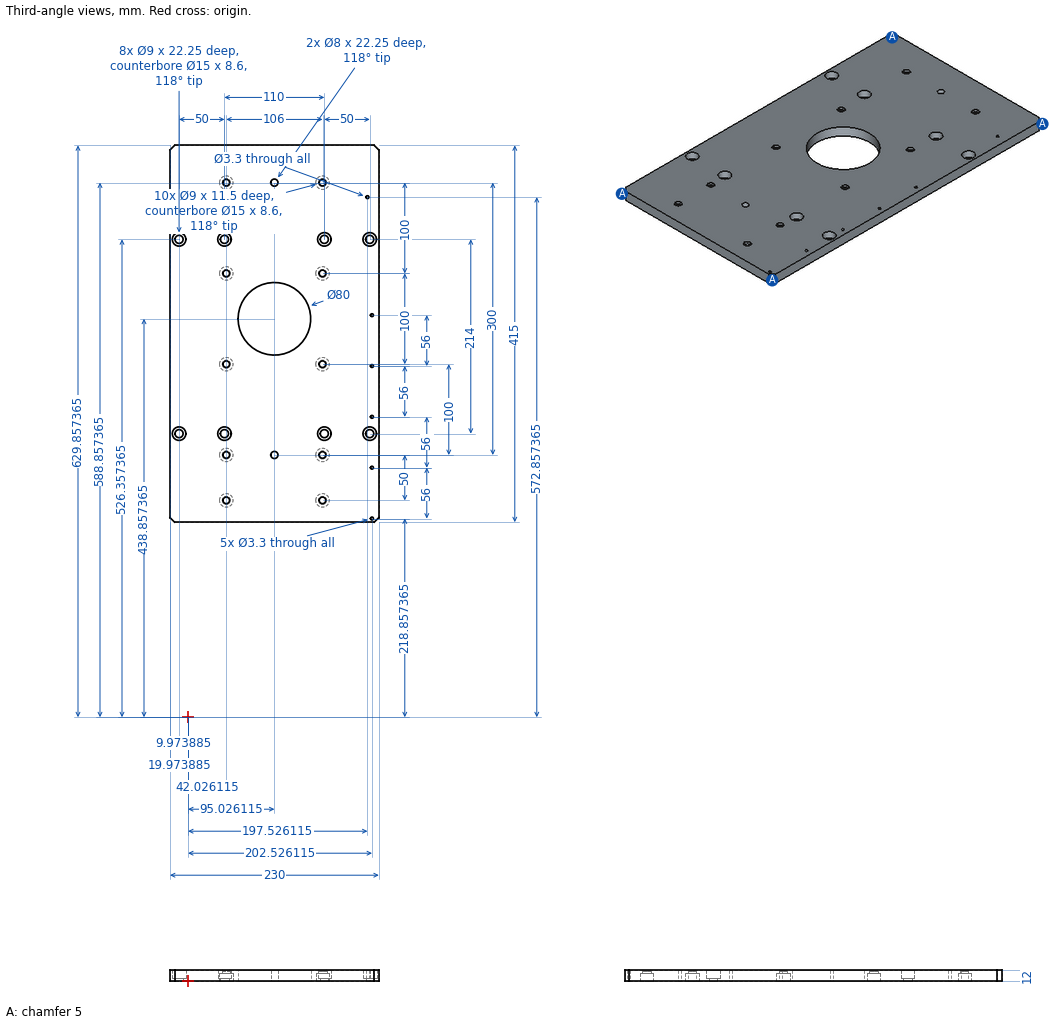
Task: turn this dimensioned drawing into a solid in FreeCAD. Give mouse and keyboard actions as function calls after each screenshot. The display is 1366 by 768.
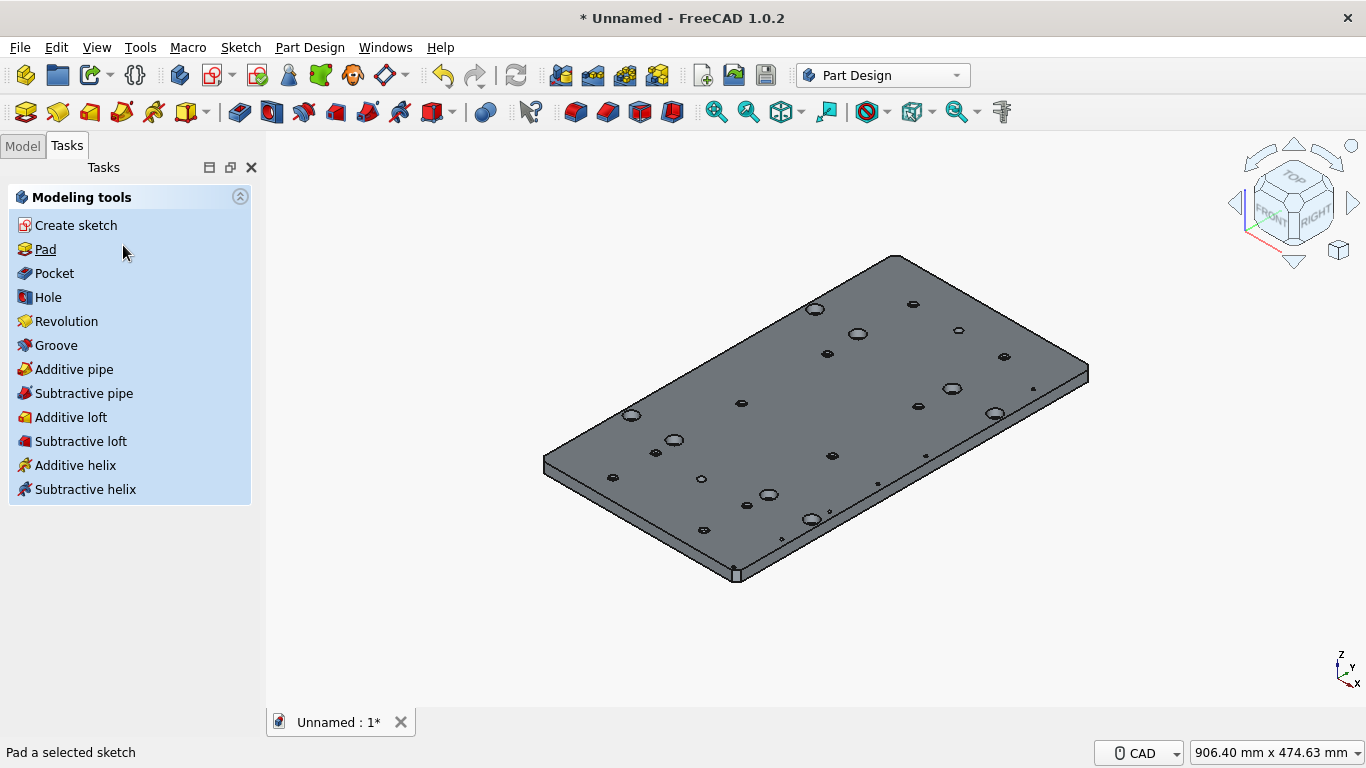
click(240, 112)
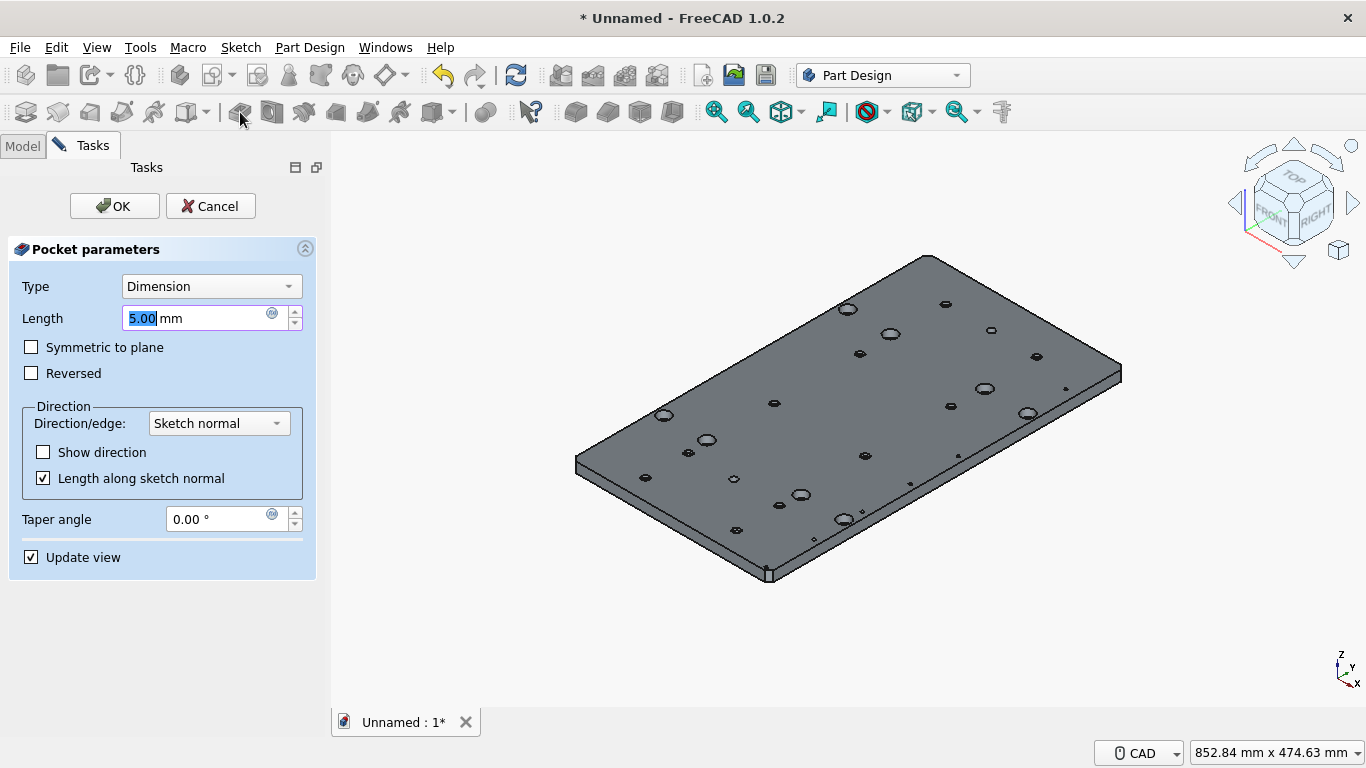
click(212, 286)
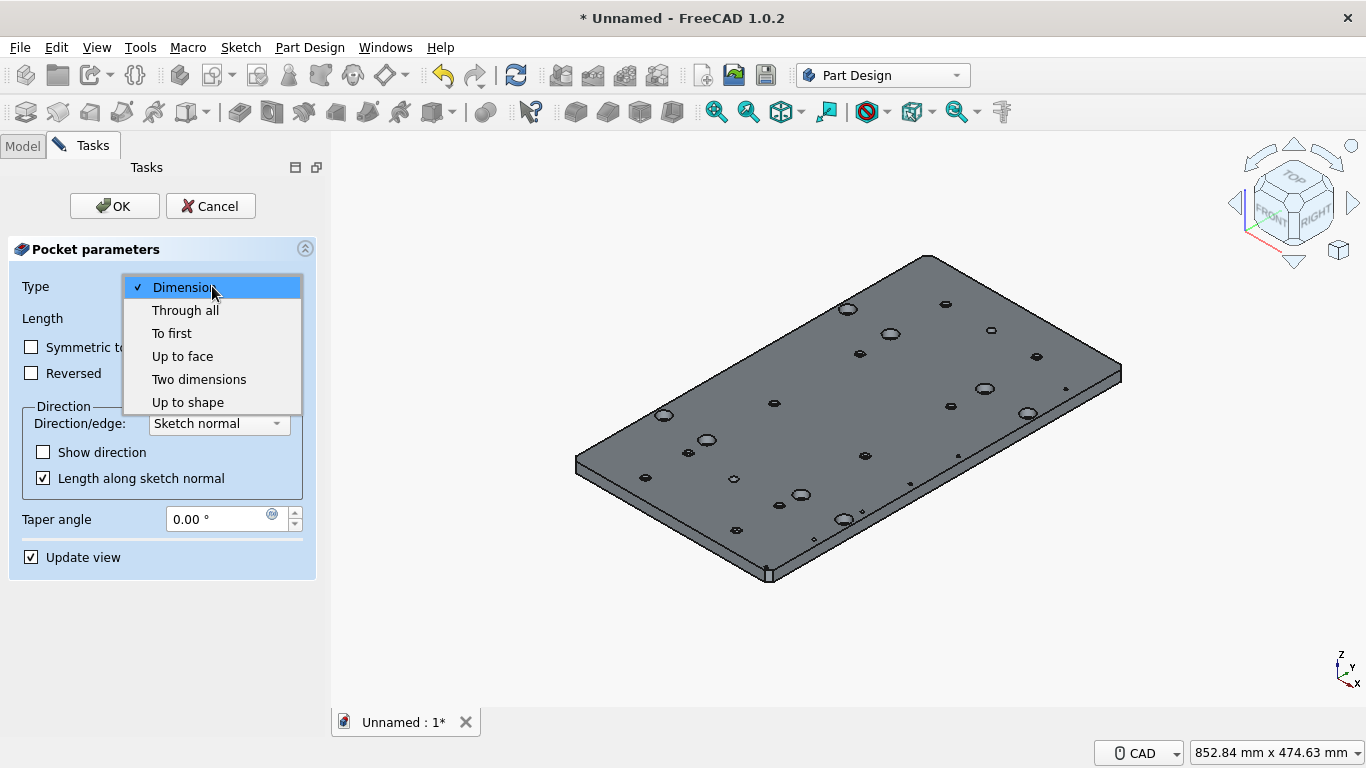
click(212, 310)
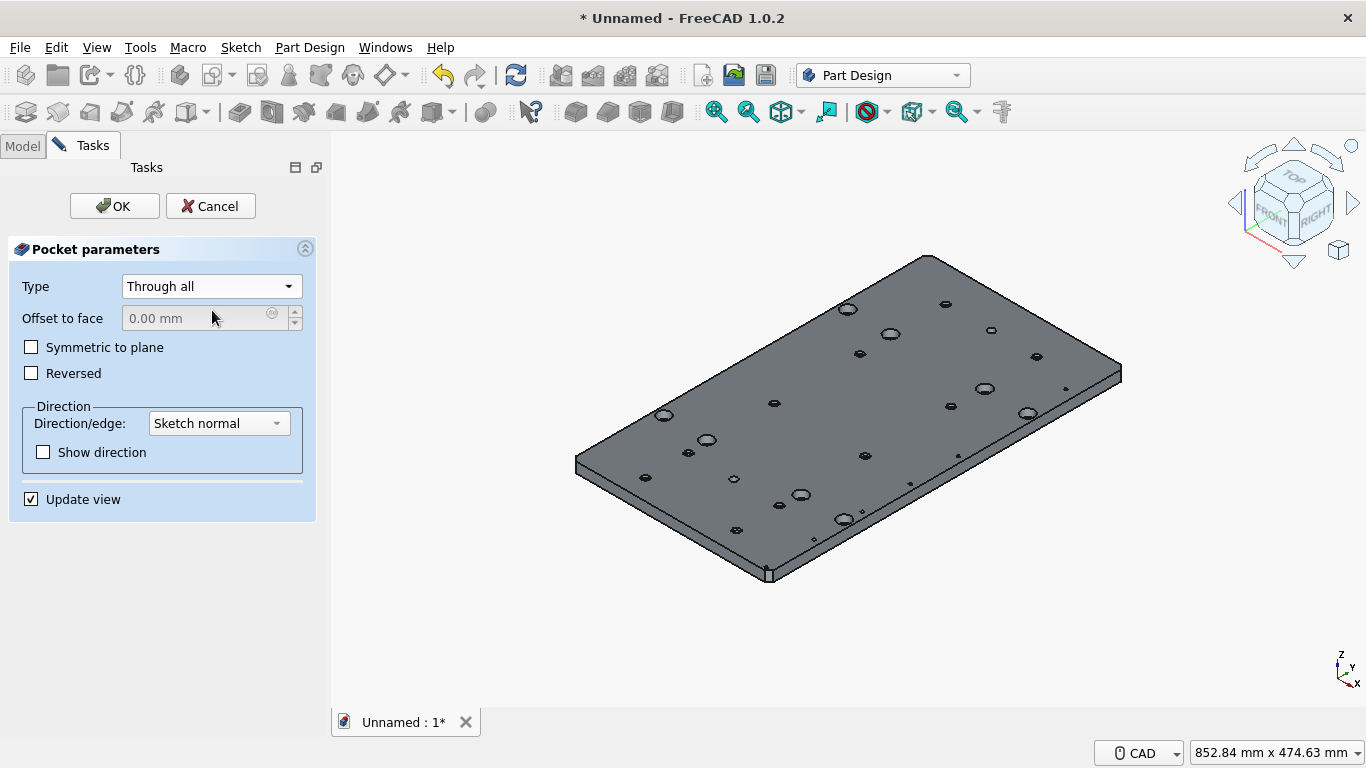
click(30, 373)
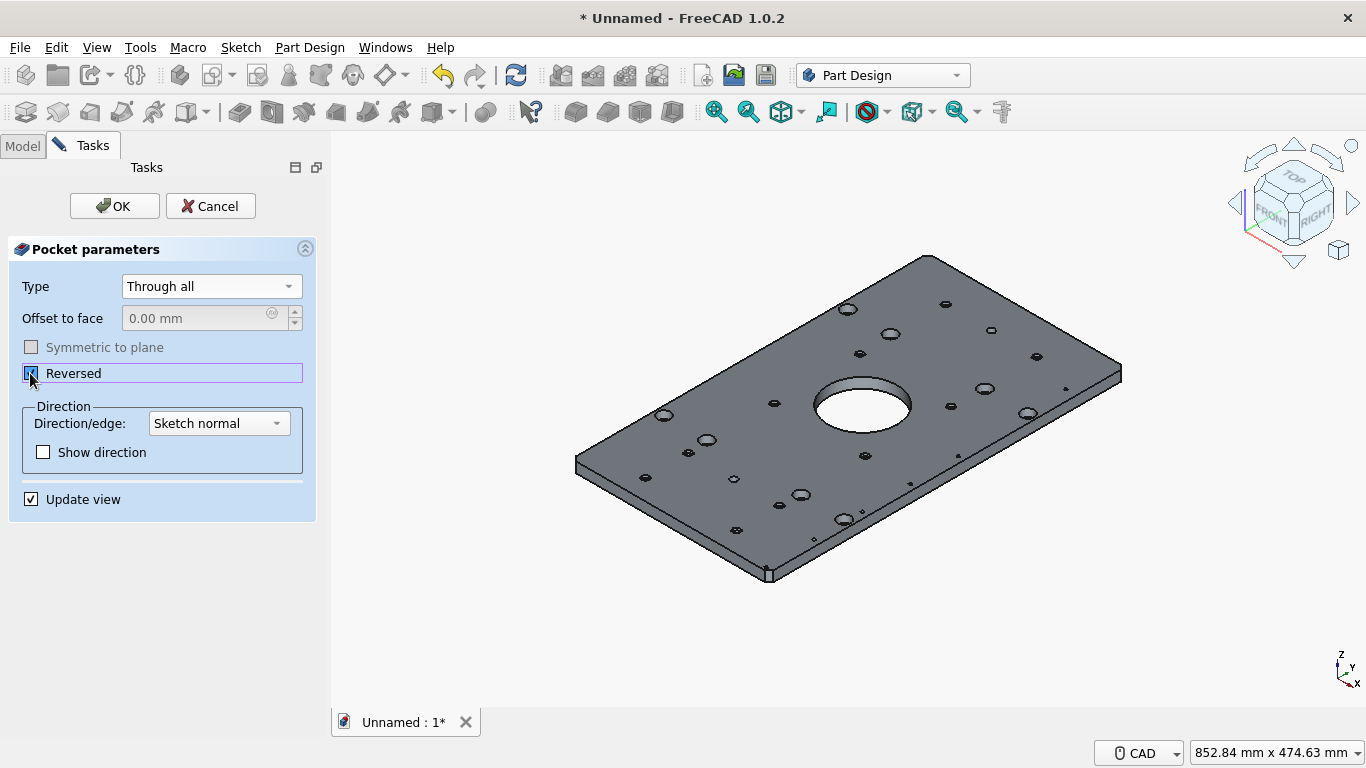
click(115, 206)